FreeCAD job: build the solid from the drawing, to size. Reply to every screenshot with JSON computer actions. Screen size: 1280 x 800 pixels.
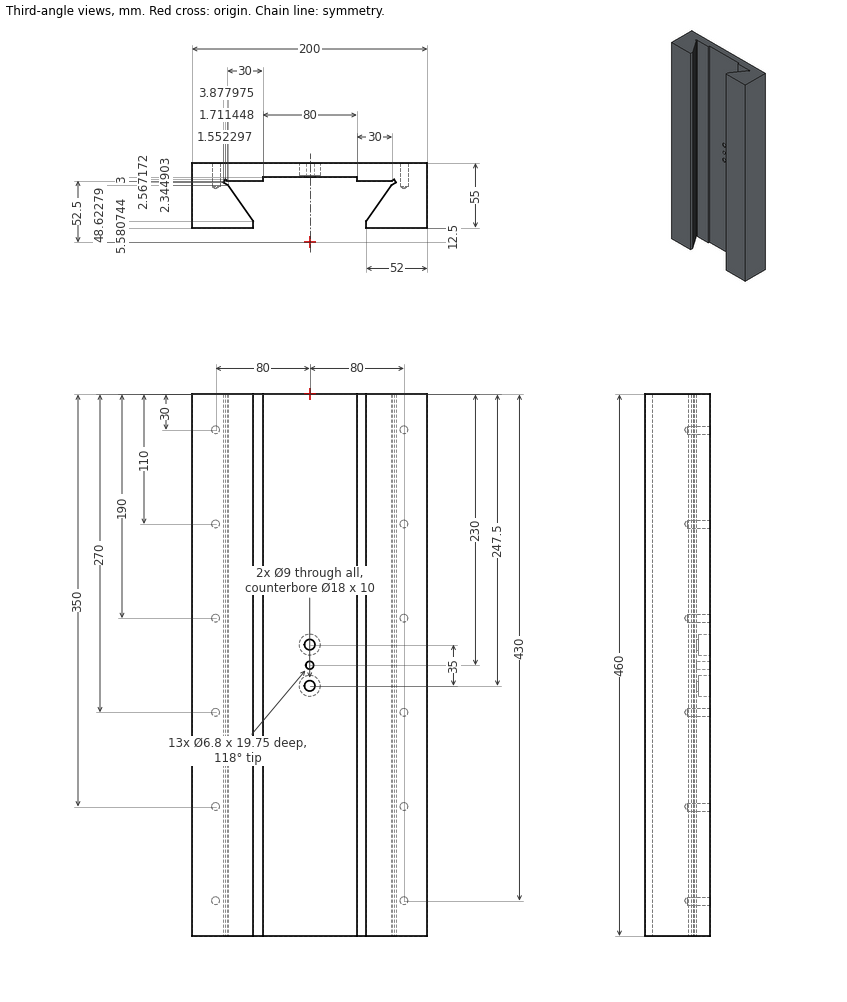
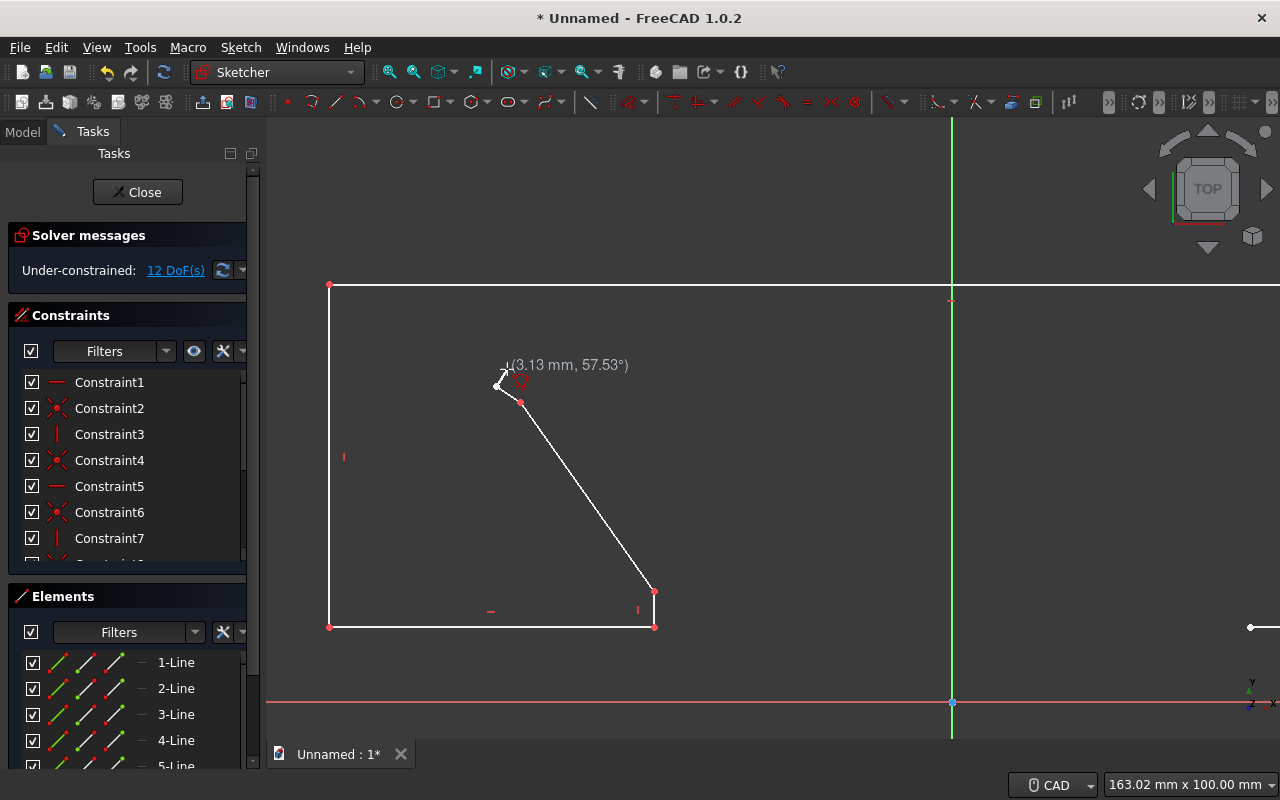
{"action": "left_click", "coordinate": [506, 369]}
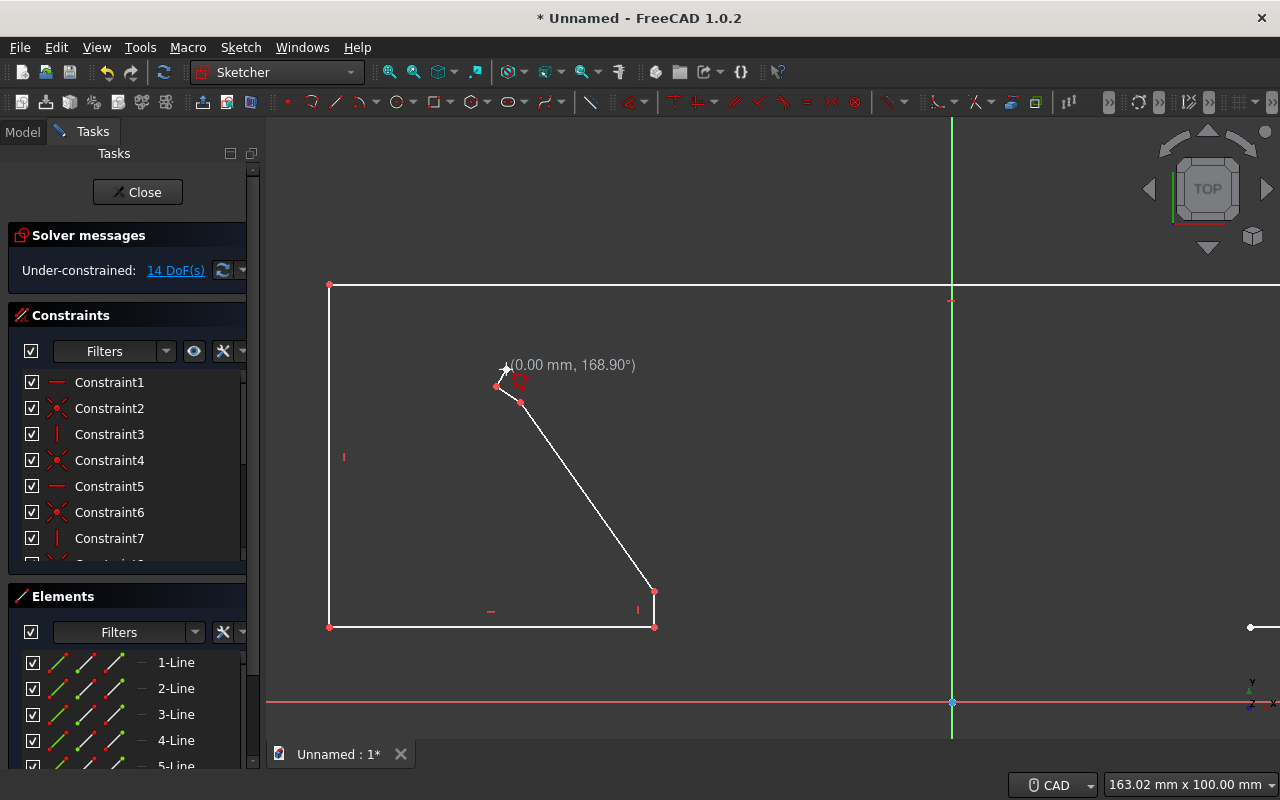
{"action": "scroll", "coordinate": [517, 376], "scroll_direction": "up", "scroll_amount": 2}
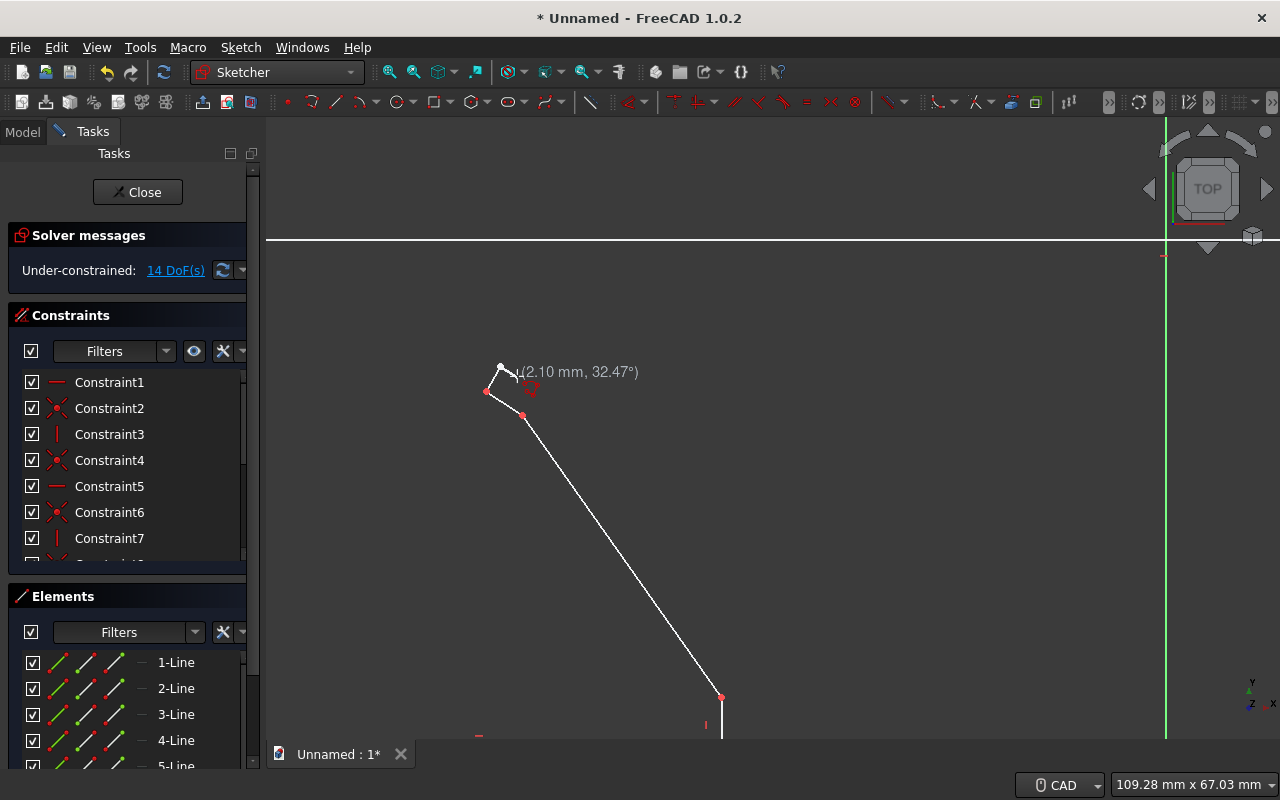
{"action": "left_click", "coordinate": [517, 375]}
{"action": "left_click", "coordinate": [795, 375]}
{"action": "left_click", "coordinate": [795, 348]}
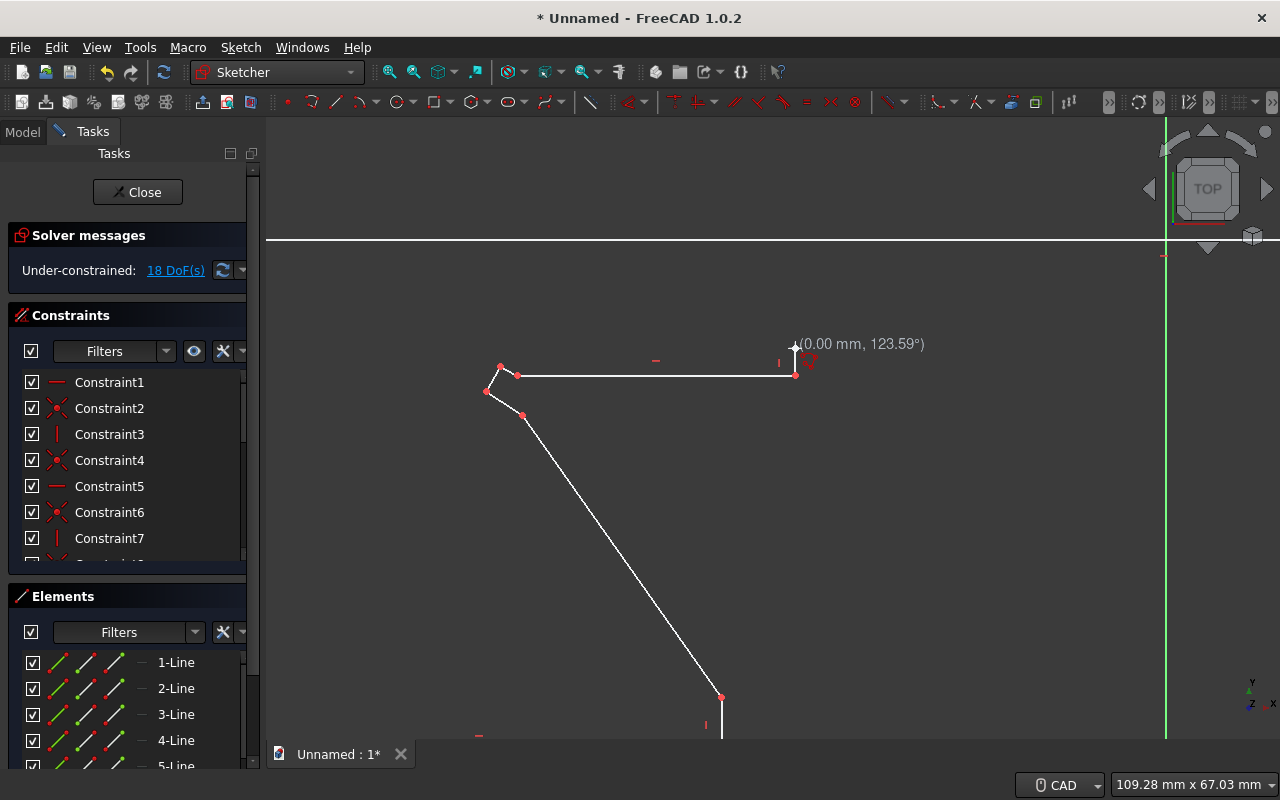
{"action": "scroll", "coordinate": [505, 376], "scroll_direction": "down", "scroll_amount": 6}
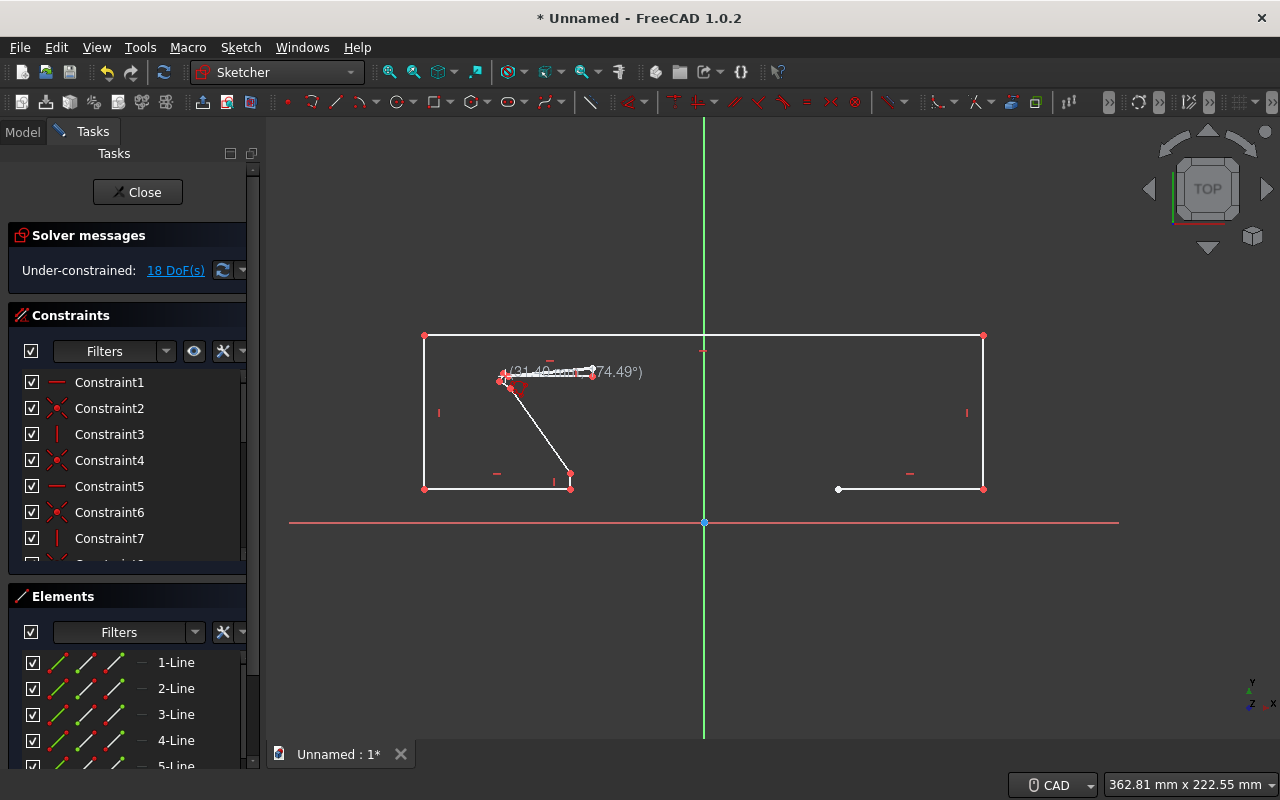
{"action": "left_click", "coordinate": [816, 368]}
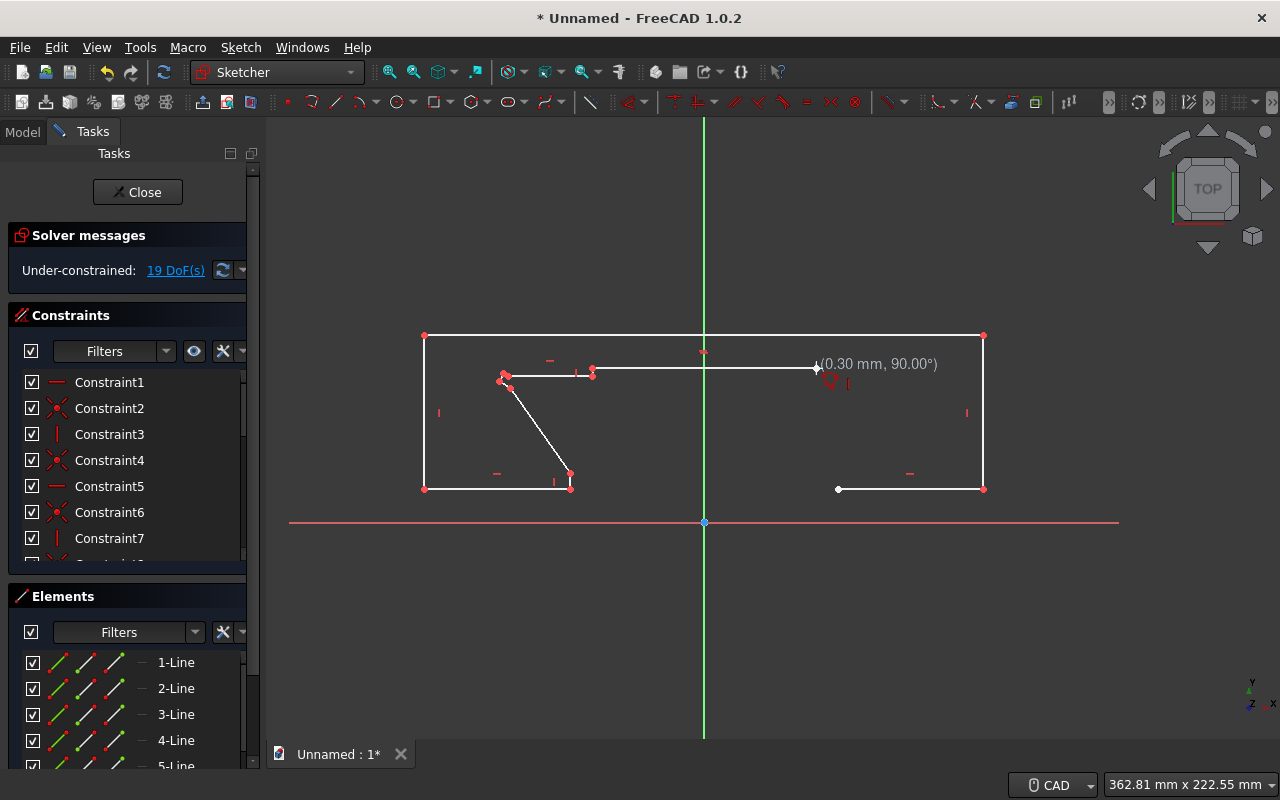
{"action": "scroll", "coordinate": [816, 376], "scroll_direction": "up", "scroll_amount": 4}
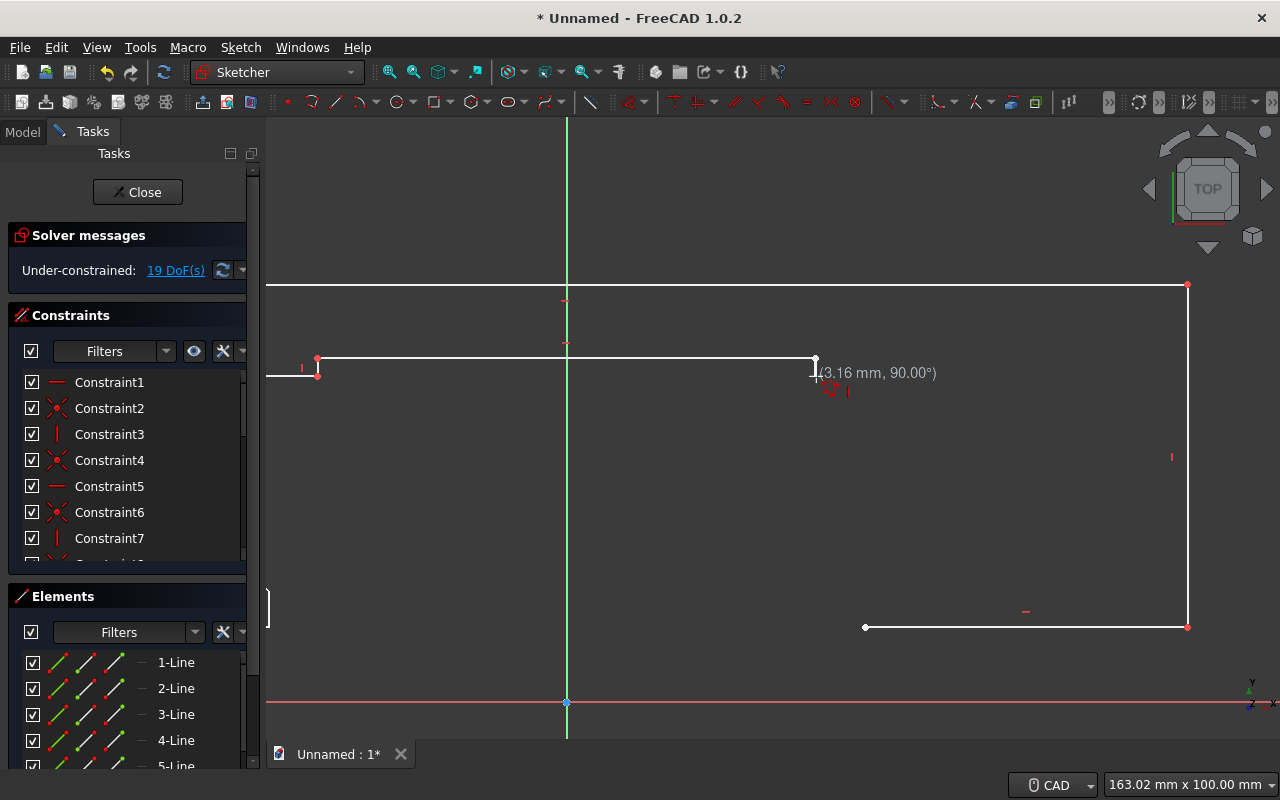
{"action": "left_click", "coordinate": [815, 376]}
{"action": "left_click", "coordinate": [1002, 376]}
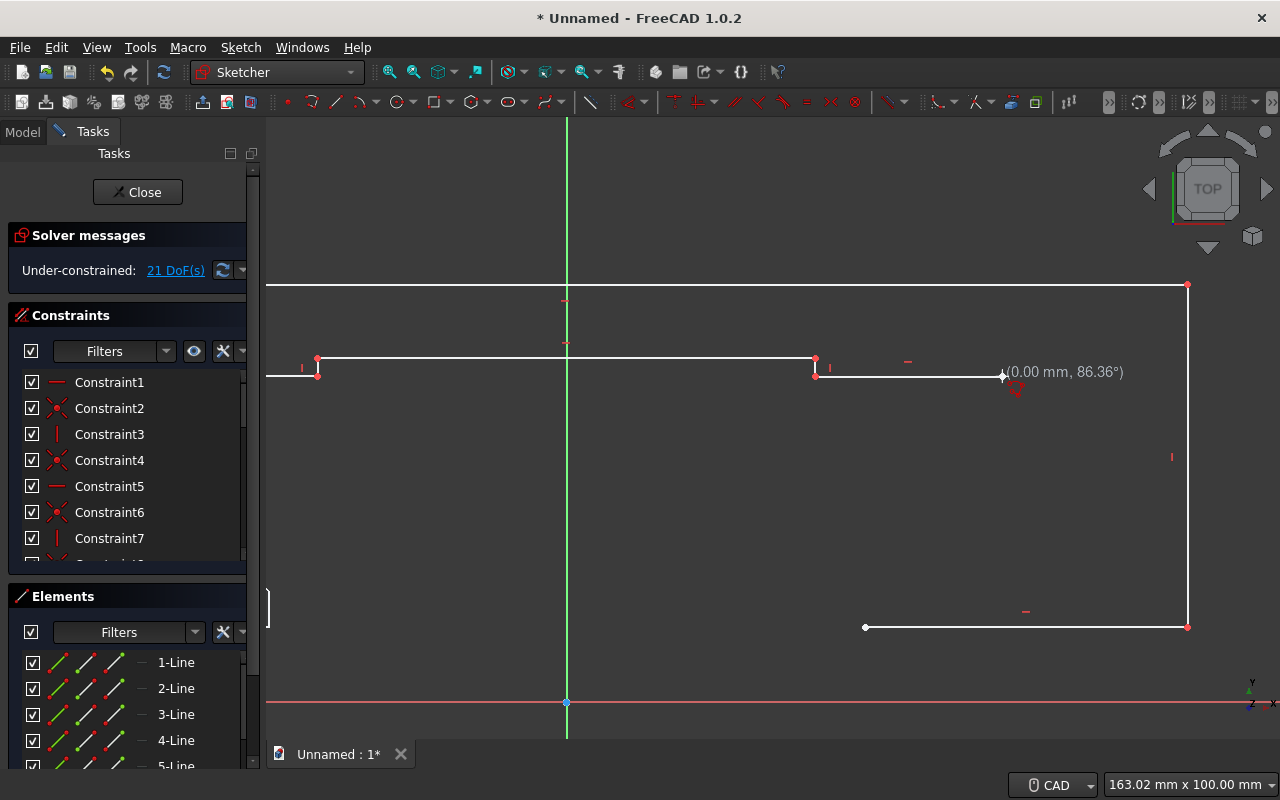
{"action": "scroll", "coordinate": [1013, 369], "scroll_direction": "up", "scroll_amount": 2}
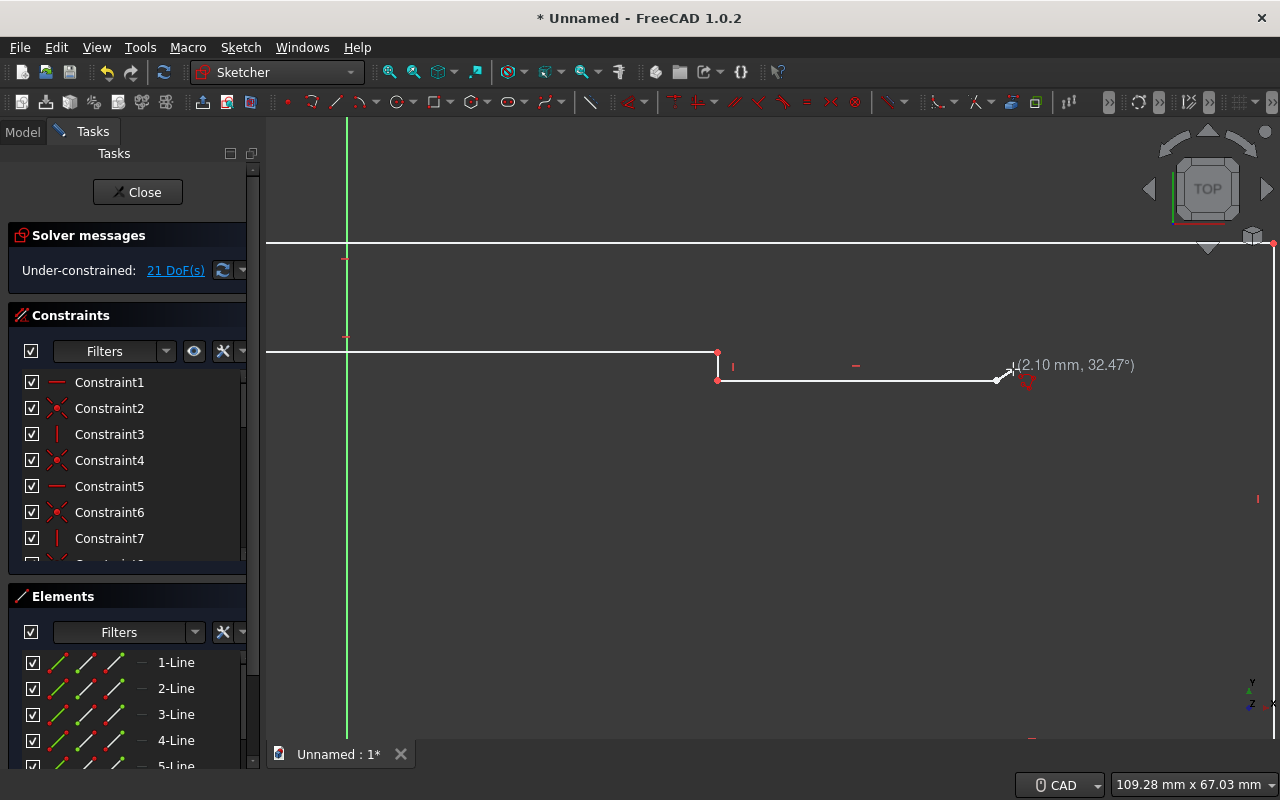
{"action": "left_click", "coordinate": [1012, 369]}
{"action": "left_click", "coordinate": [1027, 393]}
{"action": "left_click", "coordinate": [991, 415]}
{"action": "left_click", "coordinate": [792, 698]}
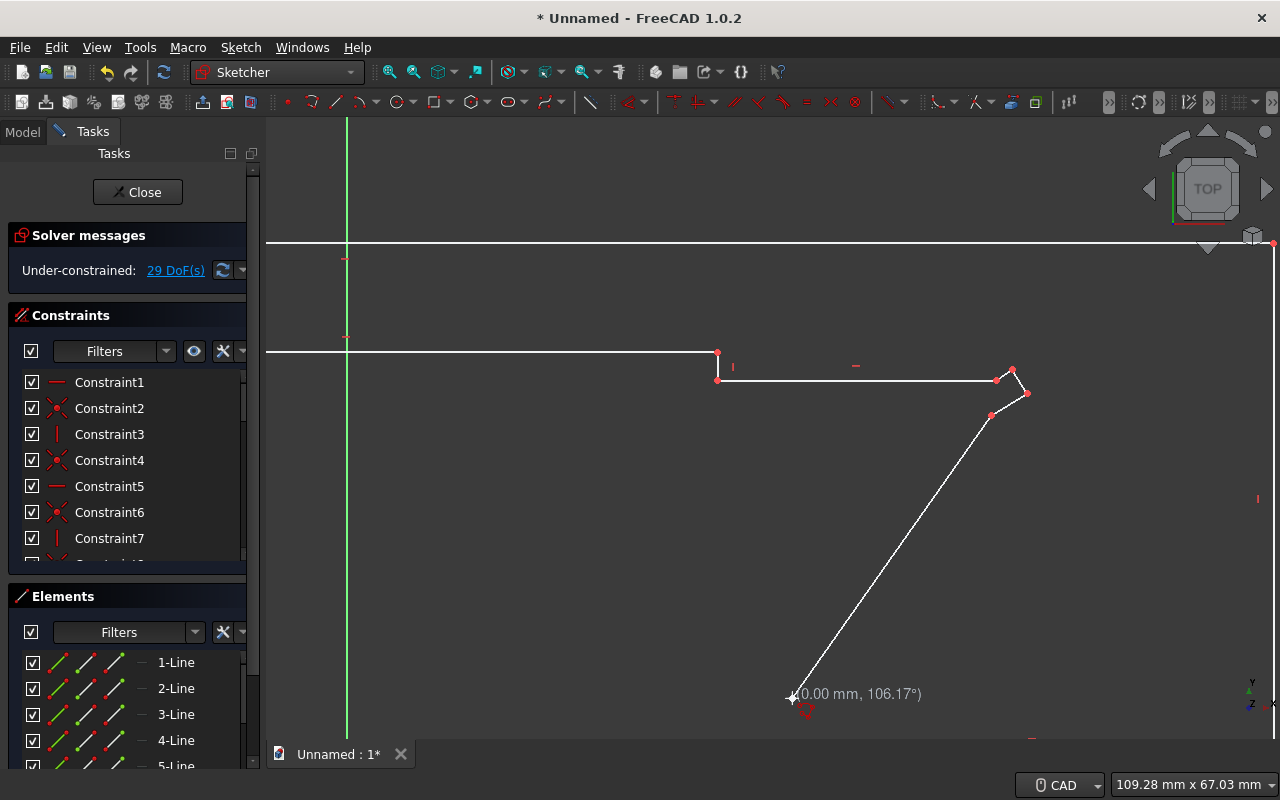
{"action": "scroll", "coordinate": [859, 374], "scroll_direction": "down", "scroll_amount": 6}